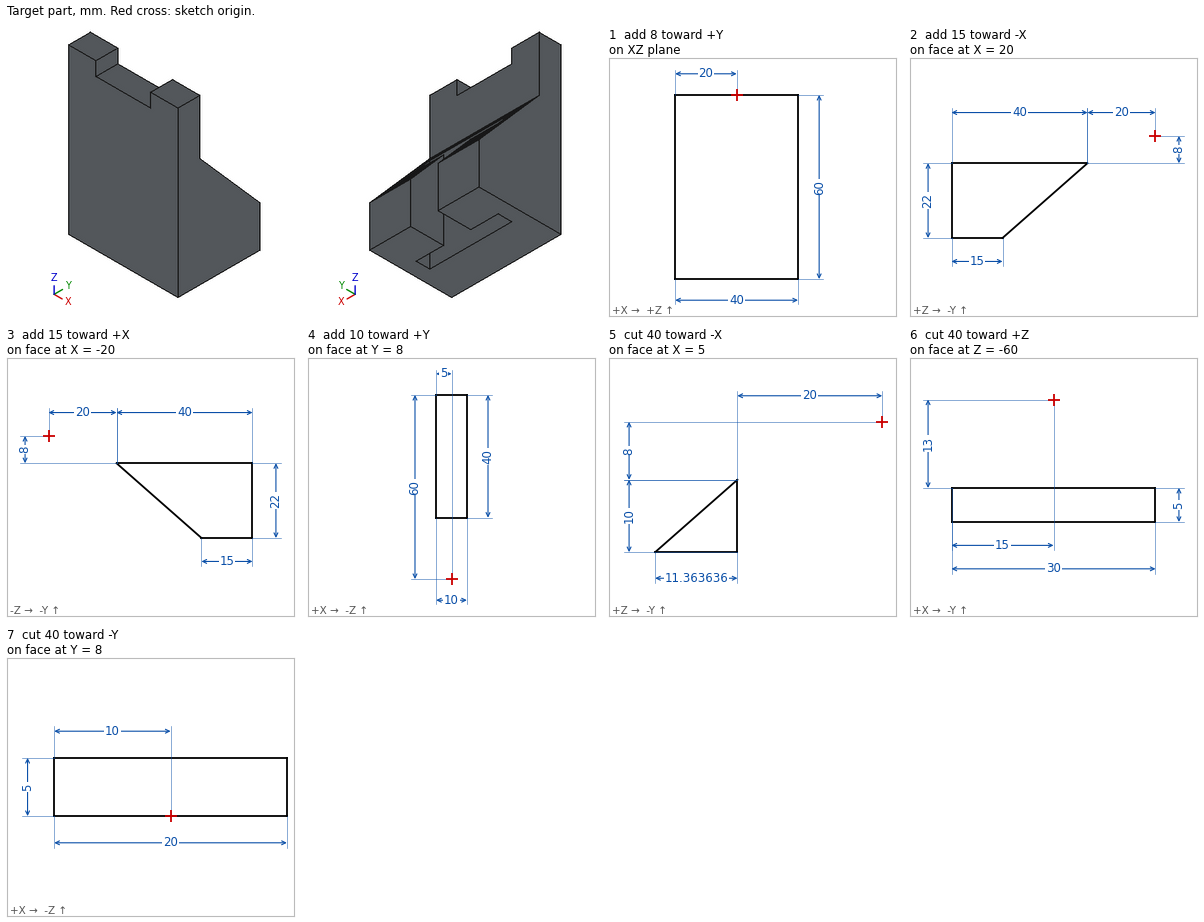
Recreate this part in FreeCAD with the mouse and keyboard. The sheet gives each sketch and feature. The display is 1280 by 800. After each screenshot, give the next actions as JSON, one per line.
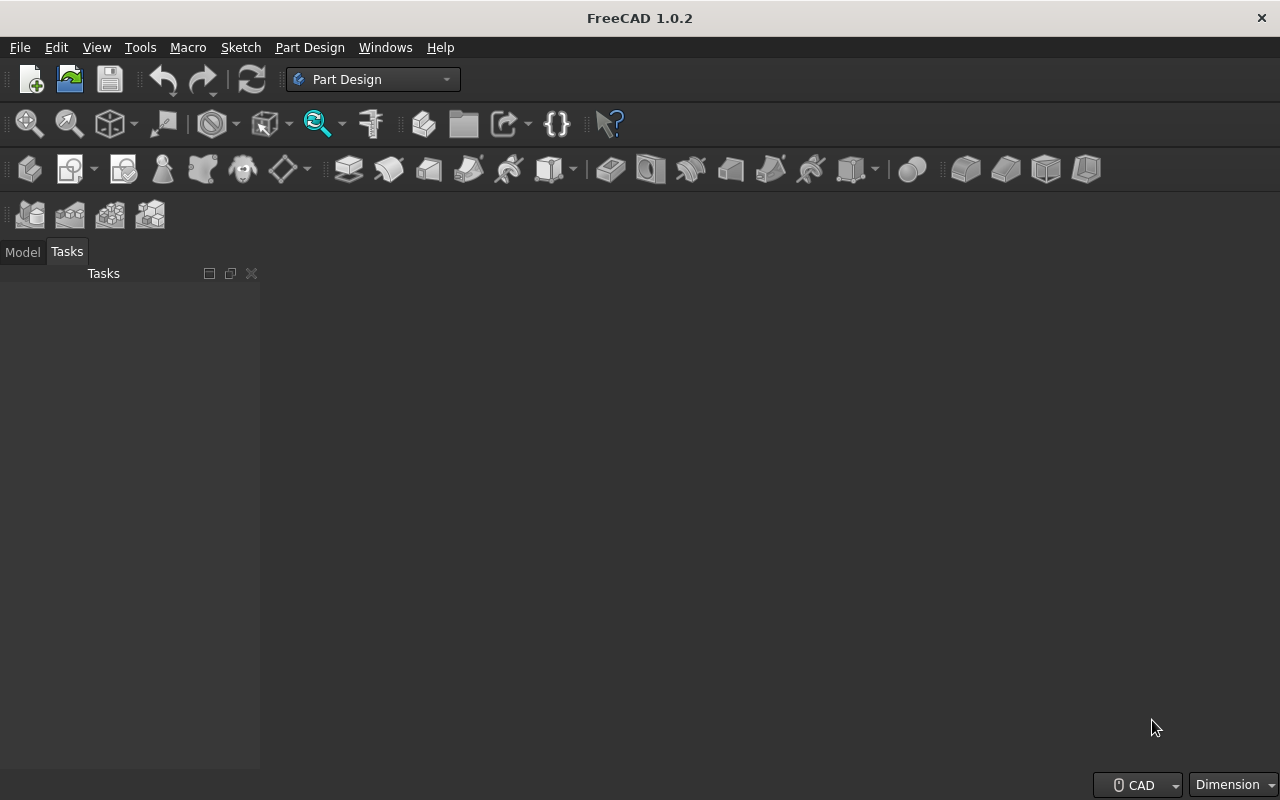
{"action": "left_click", "coordinate": [30, 80]}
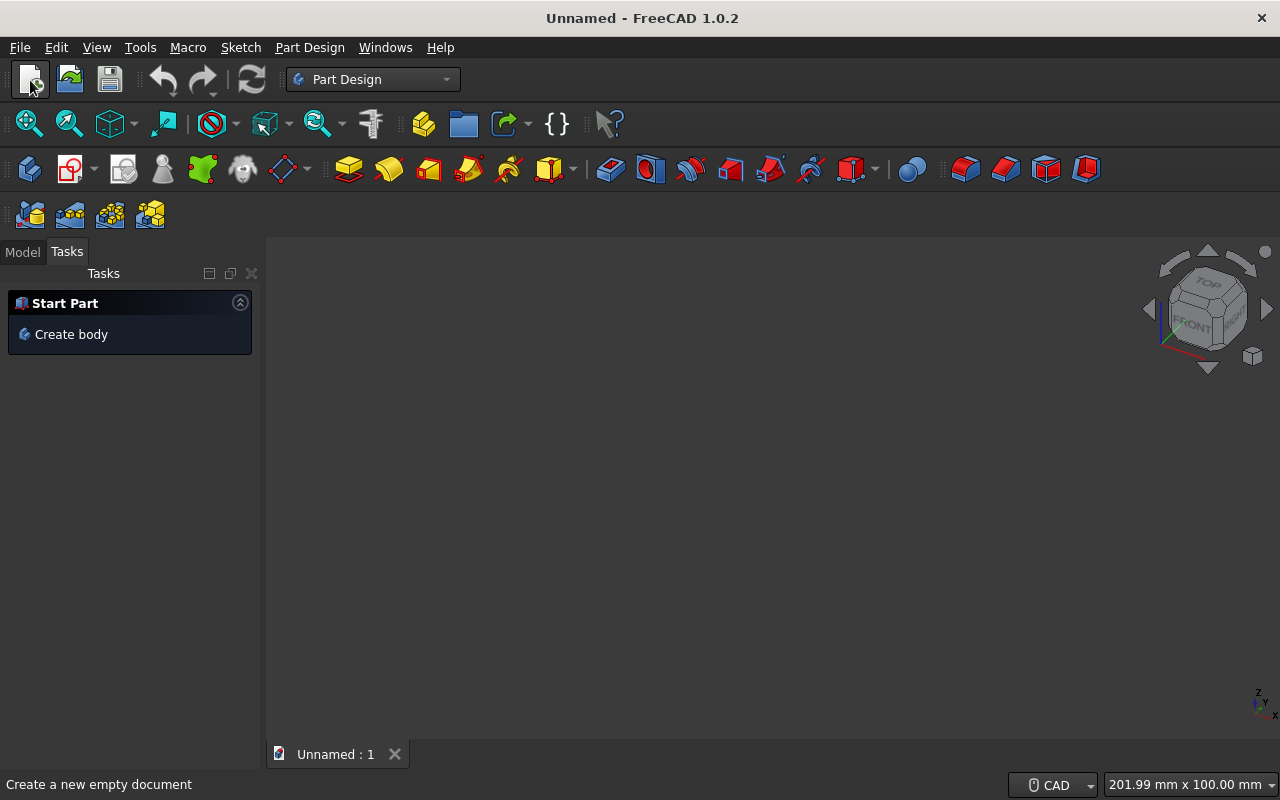
{"action": "left_click", "coordinate": [70, 170]}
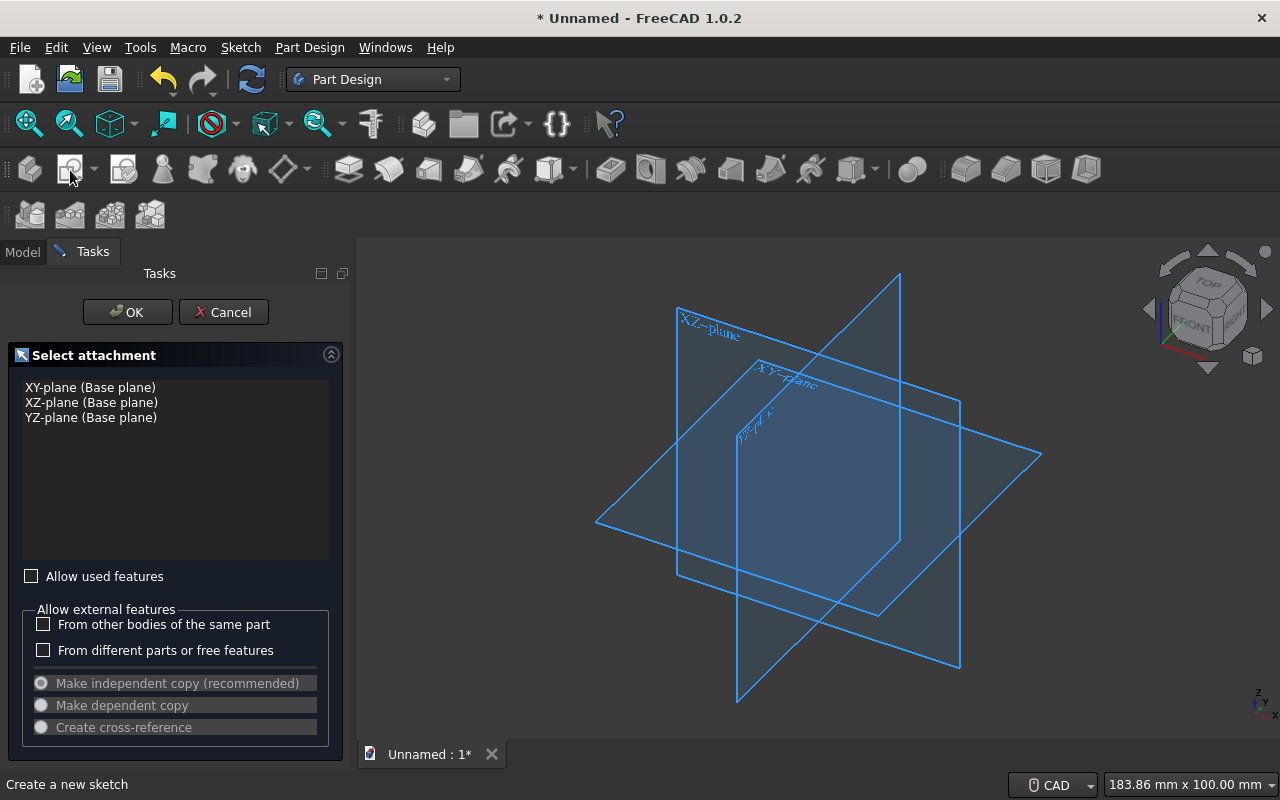
{"action": "left_click", "coordinate": [82, 402]}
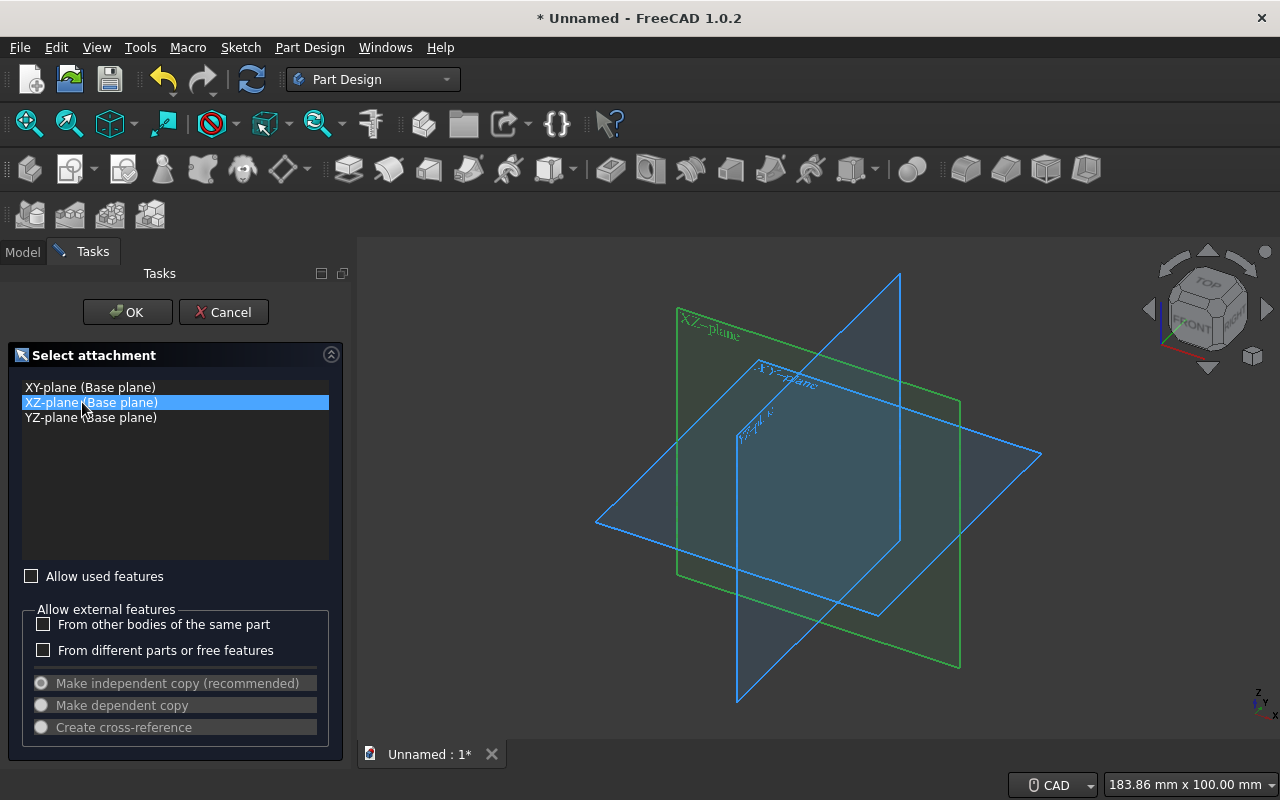
{"action": "left_click", "coordinate": [128, 312]}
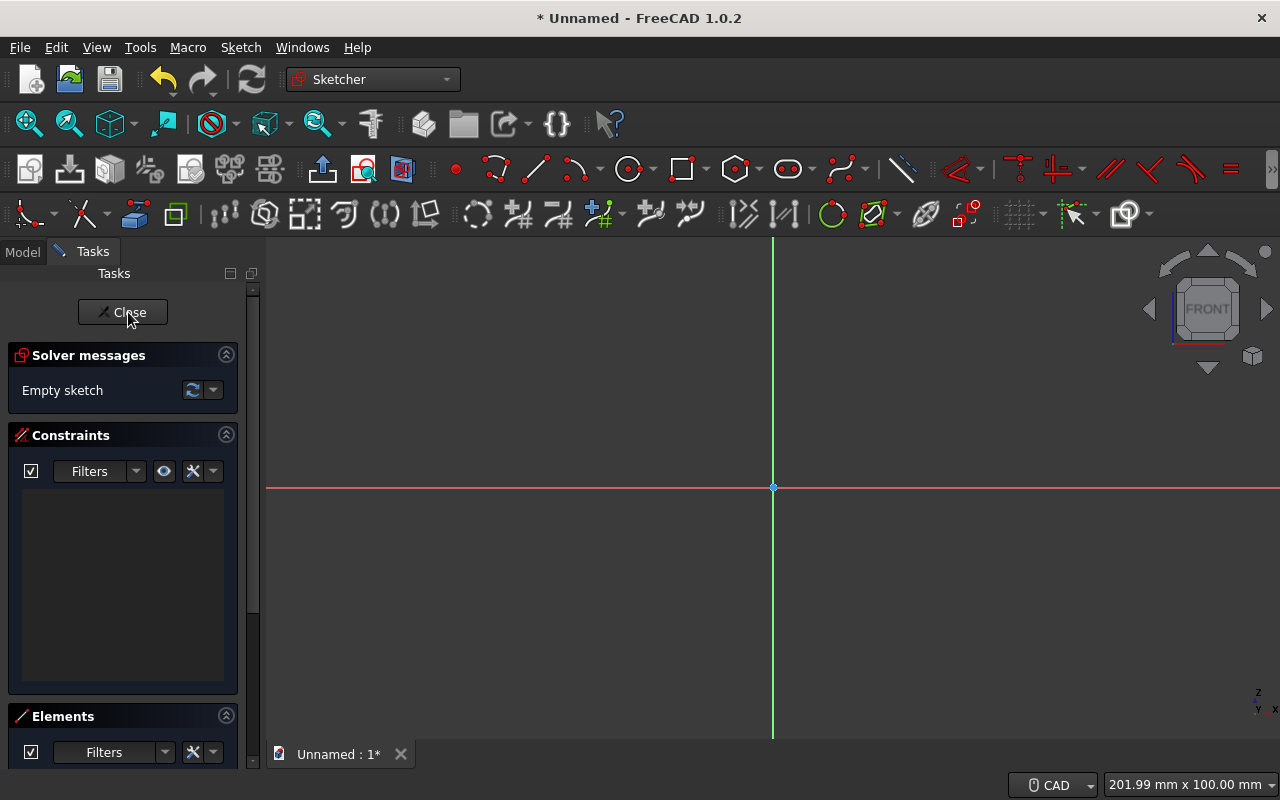
{"action": "scroll", "coordinate": [565, 265], "scroll_direction": "down", "scroll_amount": 2}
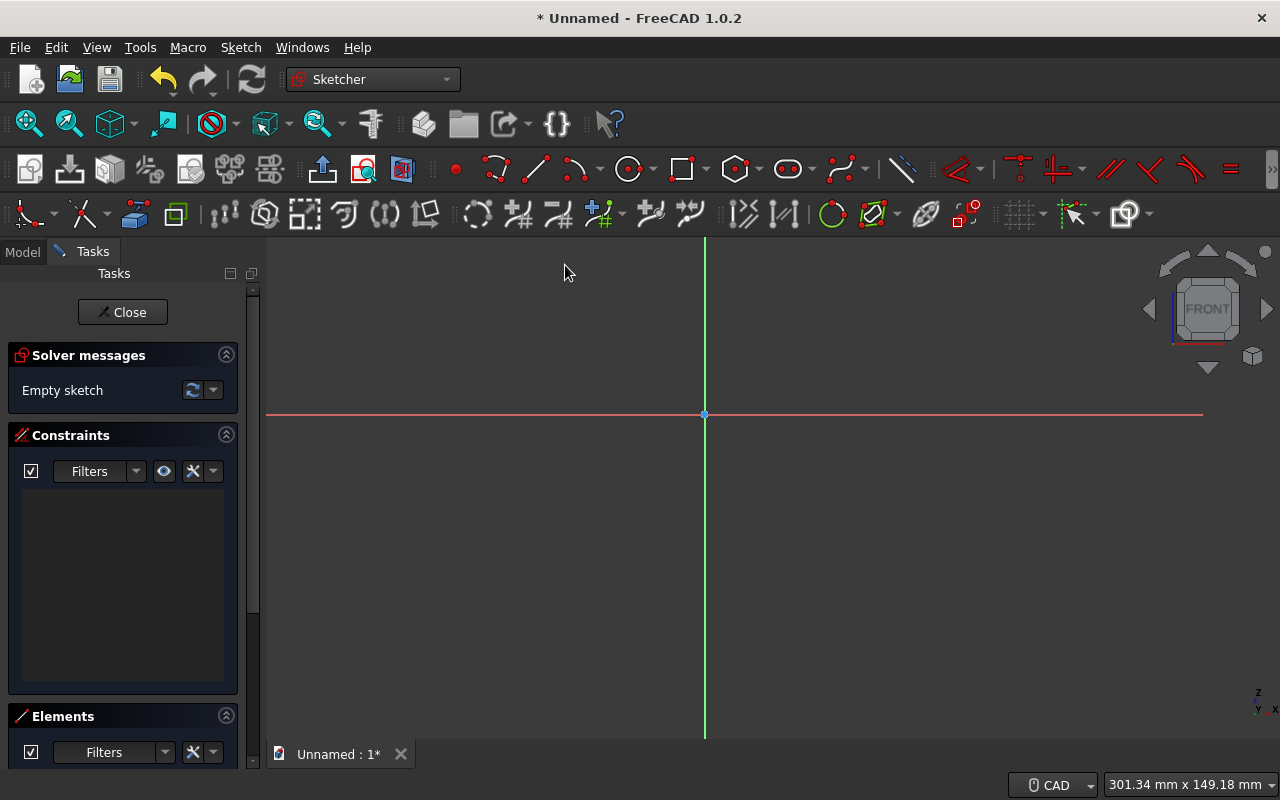
{"action": "scroll", "coordinate": [705, 571], "scroll_direction": "up", "scroll_amount": 2}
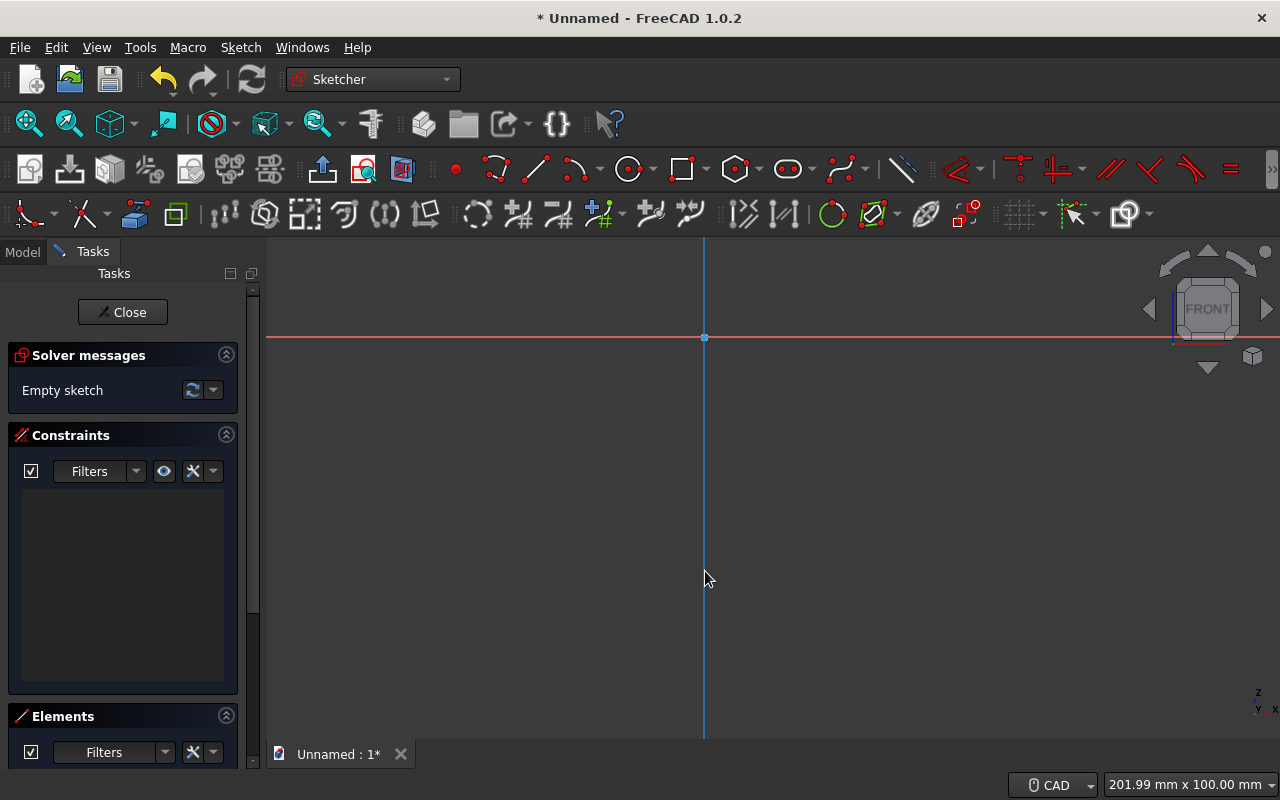
{"action": "left_click", "coordinate": [682, 170]}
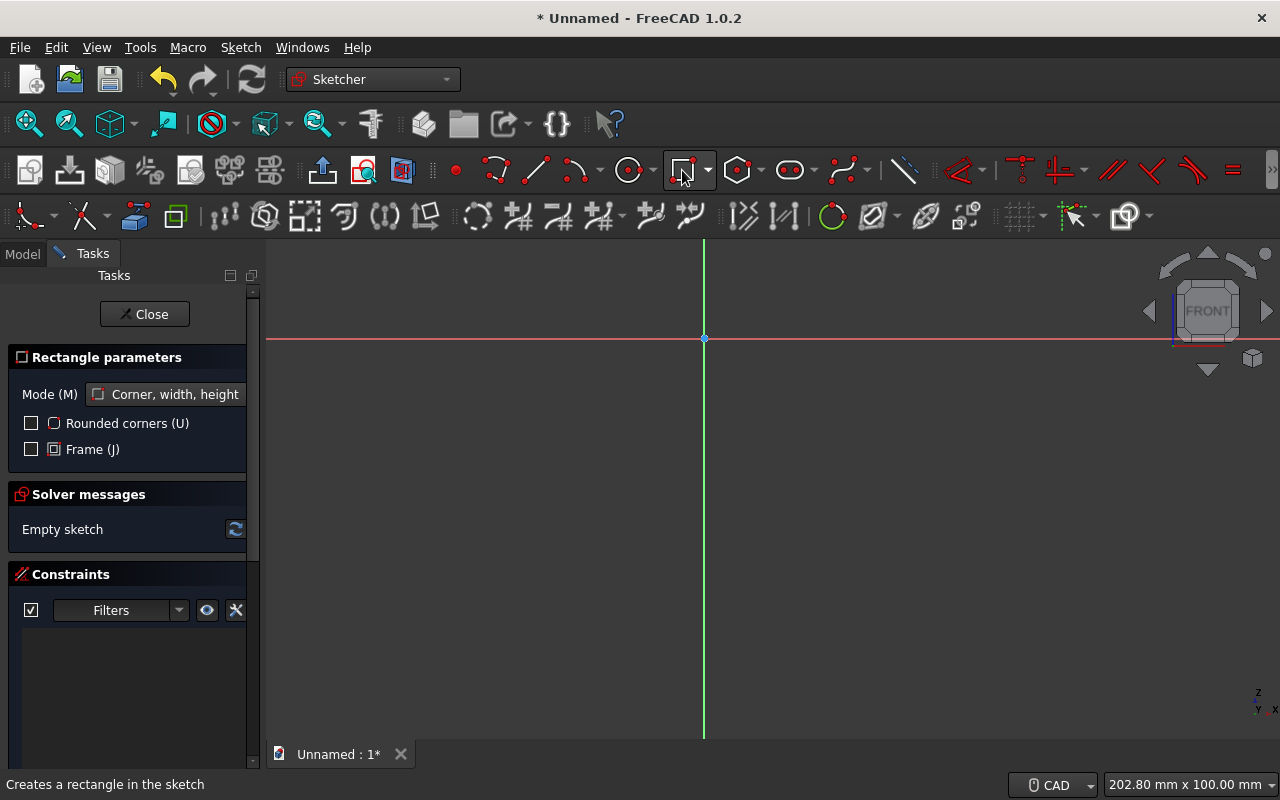
{"action": "left_click", "coordinate": [604, 339]}
{"action": "mouse_move", "coordinate": [804, 639]}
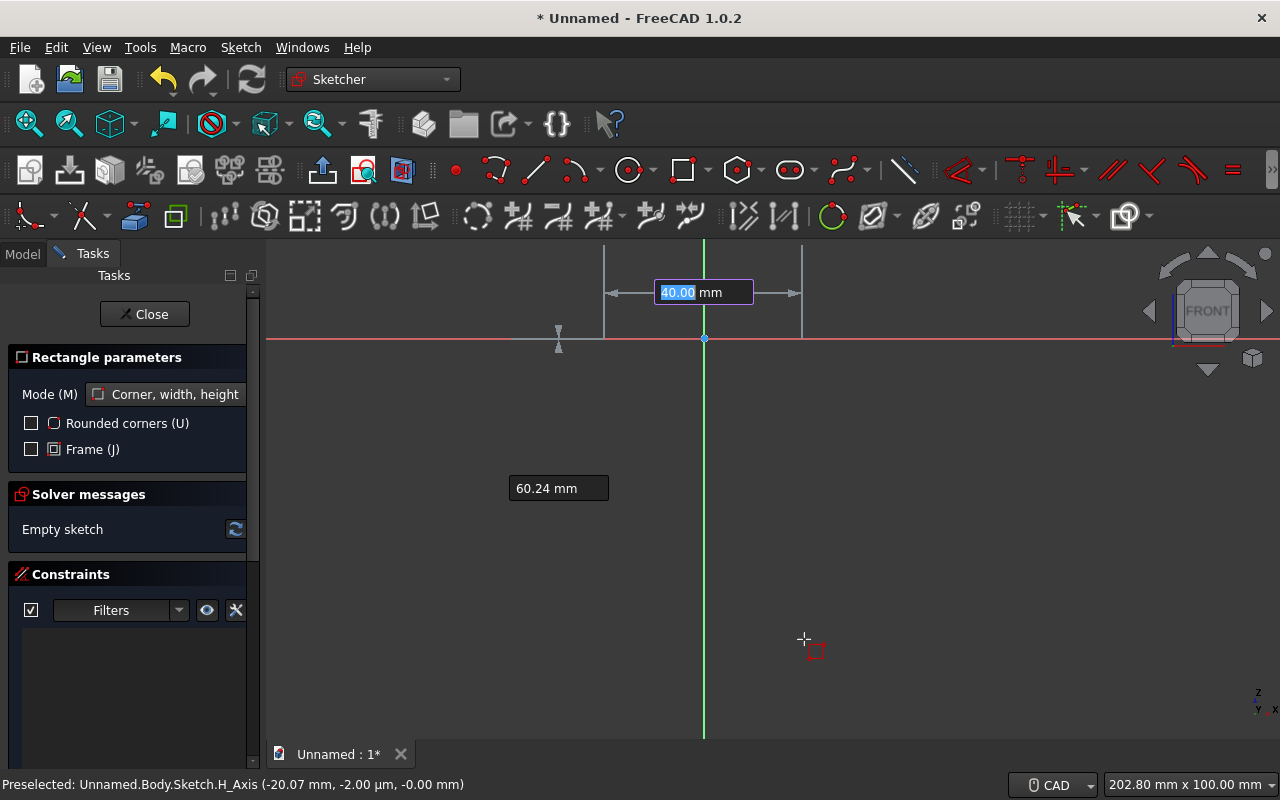
{"action": "type", "text": "40"}
{"action": "key", "text": "Tab"}
{"action": "type", "text": "60"}
{"action": "key", "text": "Return"}
{"action": "key", "text": "Escape"}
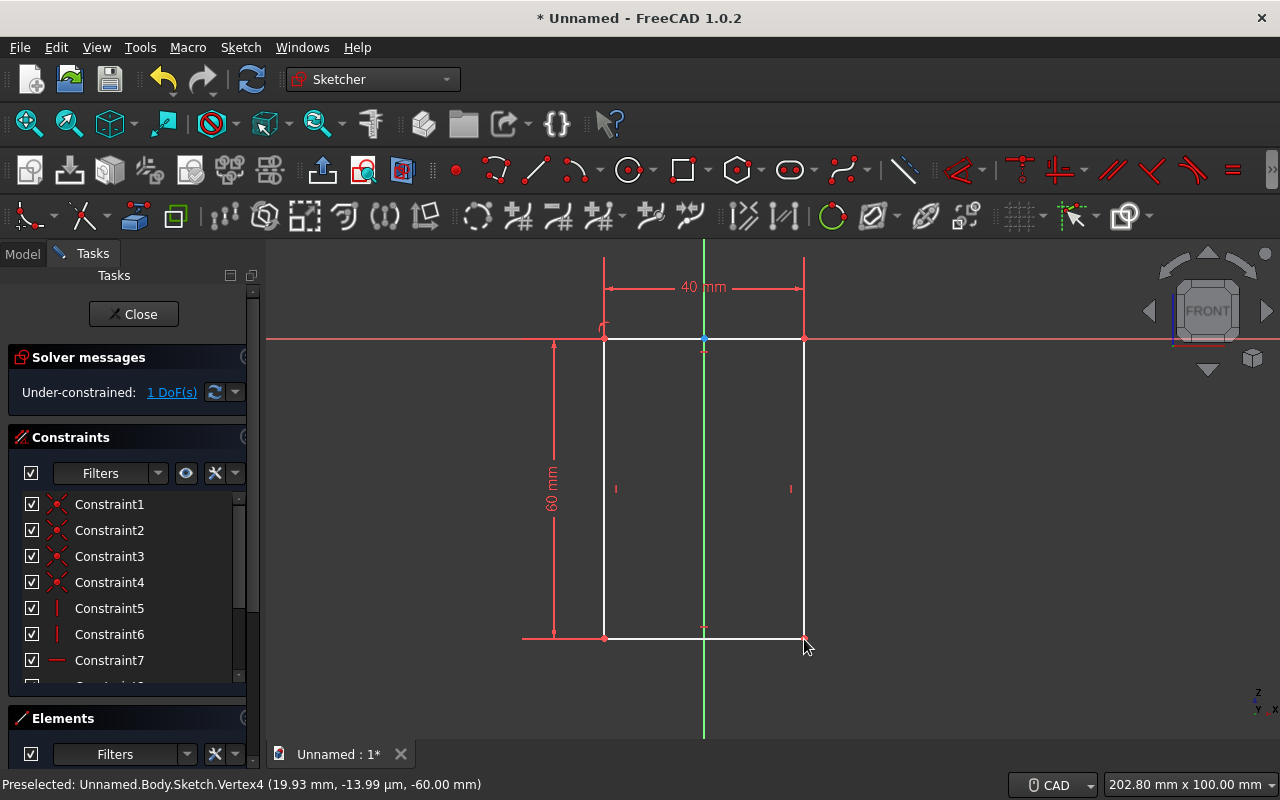
{"action": "left_click", "coordinate": [604, 339]}